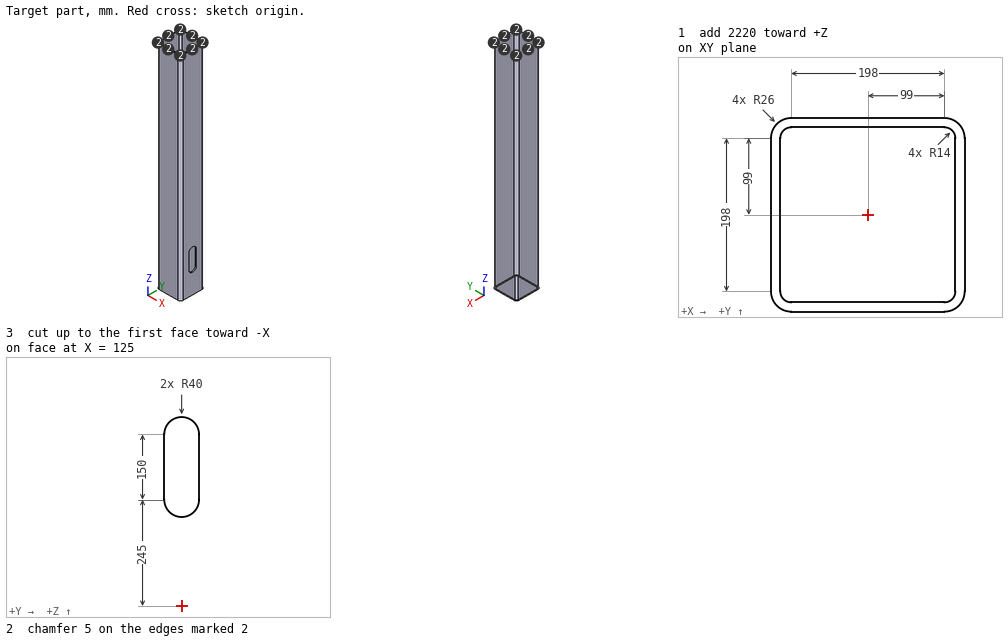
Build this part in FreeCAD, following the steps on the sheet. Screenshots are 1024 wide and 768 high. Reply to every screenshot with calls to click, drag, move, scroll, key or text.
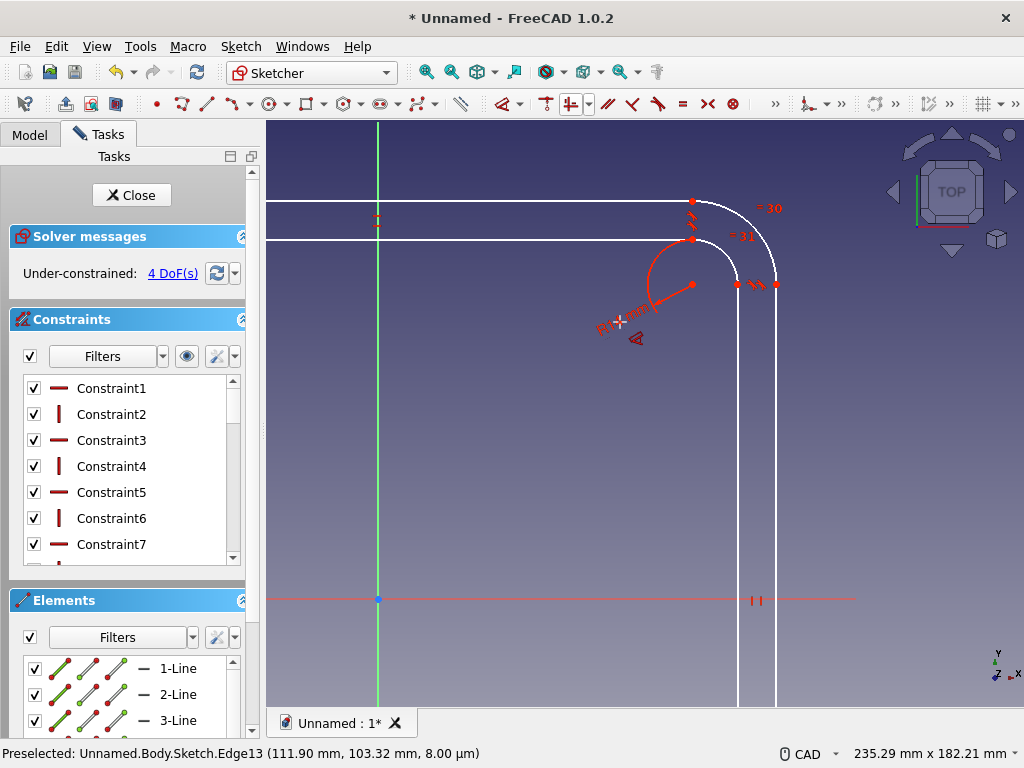
click(503, 201)
click(493, 167)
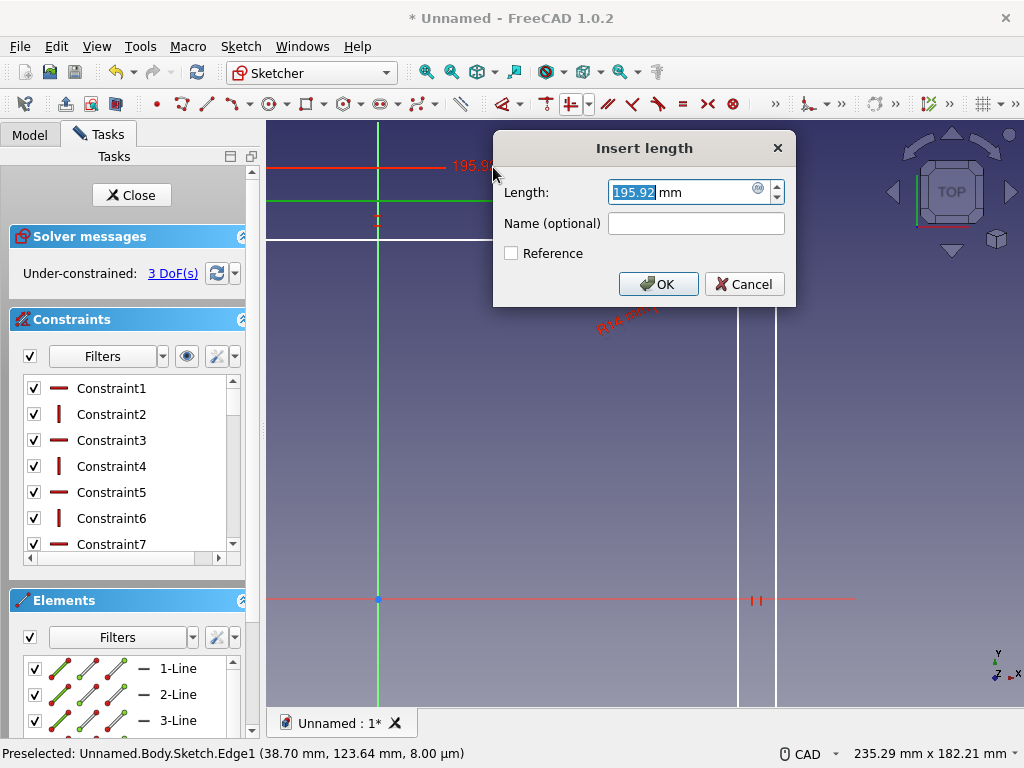
text(198)
key(Return)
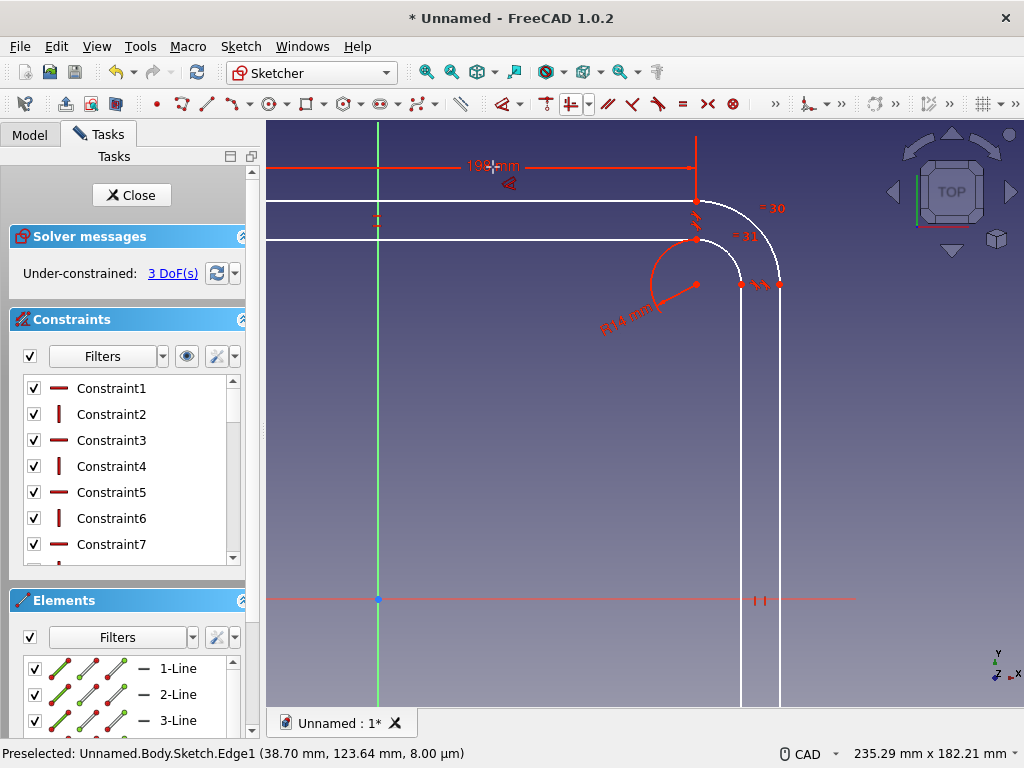
scroll(738, 262, down, 4)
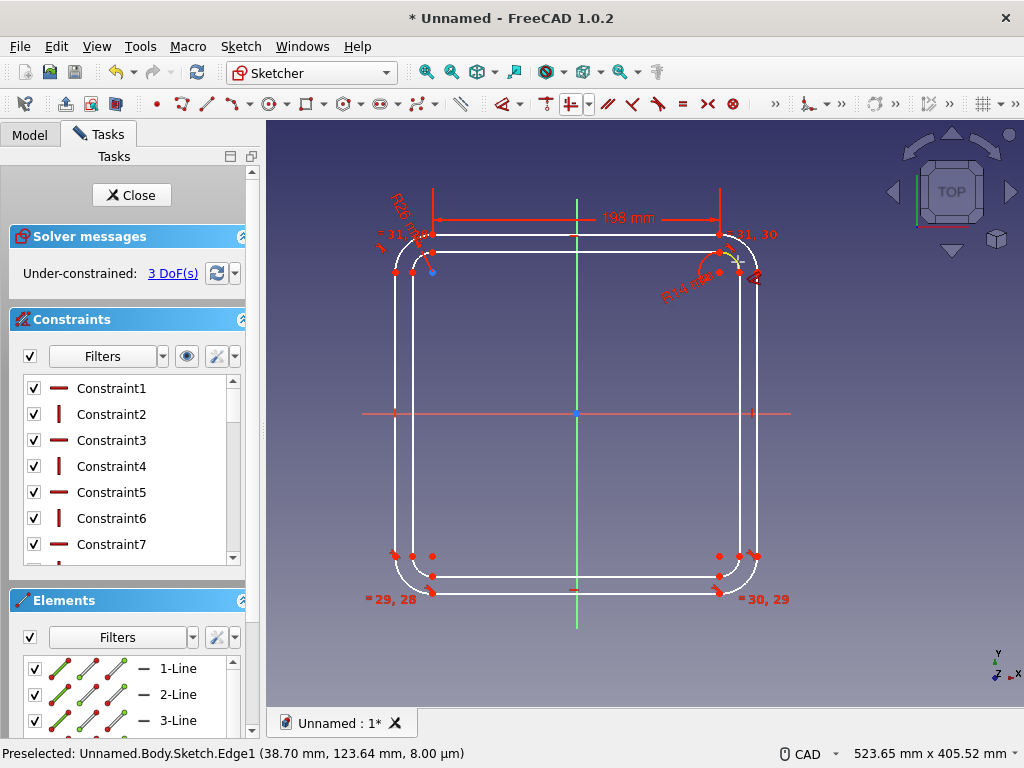
click(395, 358)
click(361, 349)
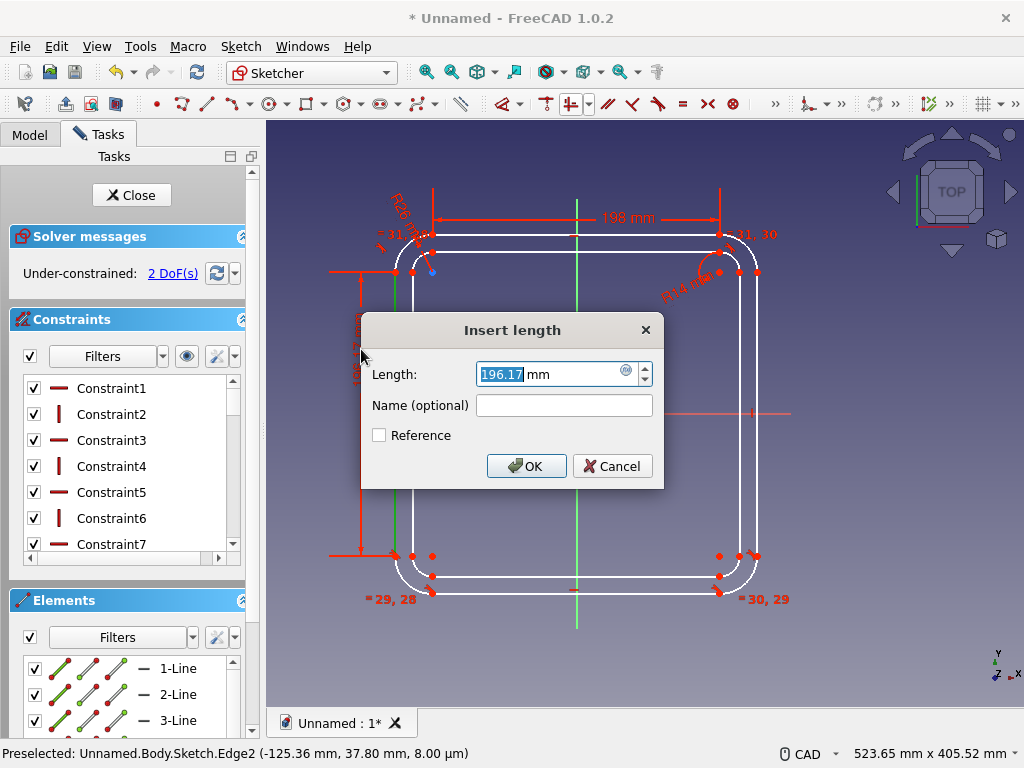
text(198)
key(Return)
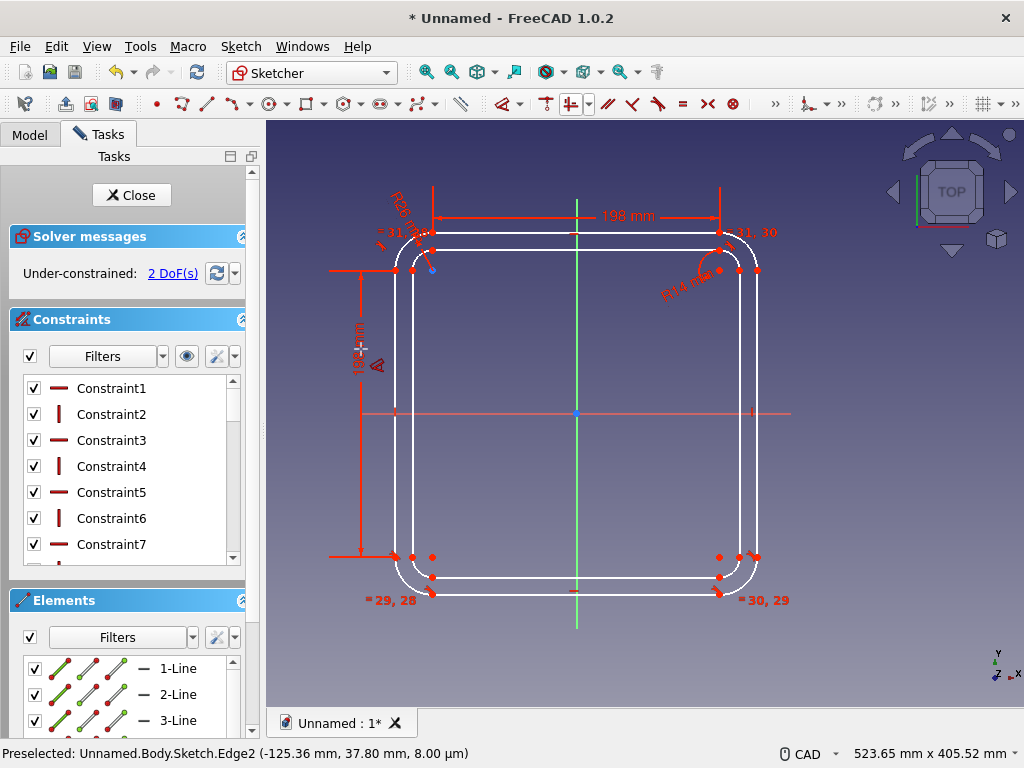
click(720, 233)
click(648, 199)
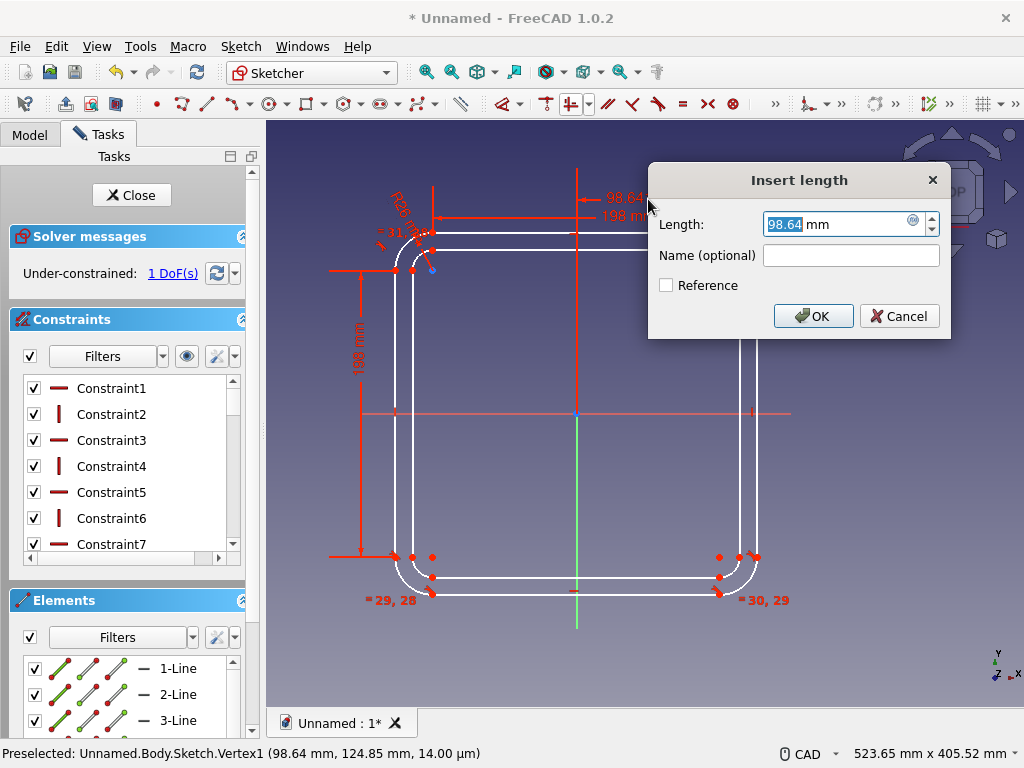
text(99)
key(Return)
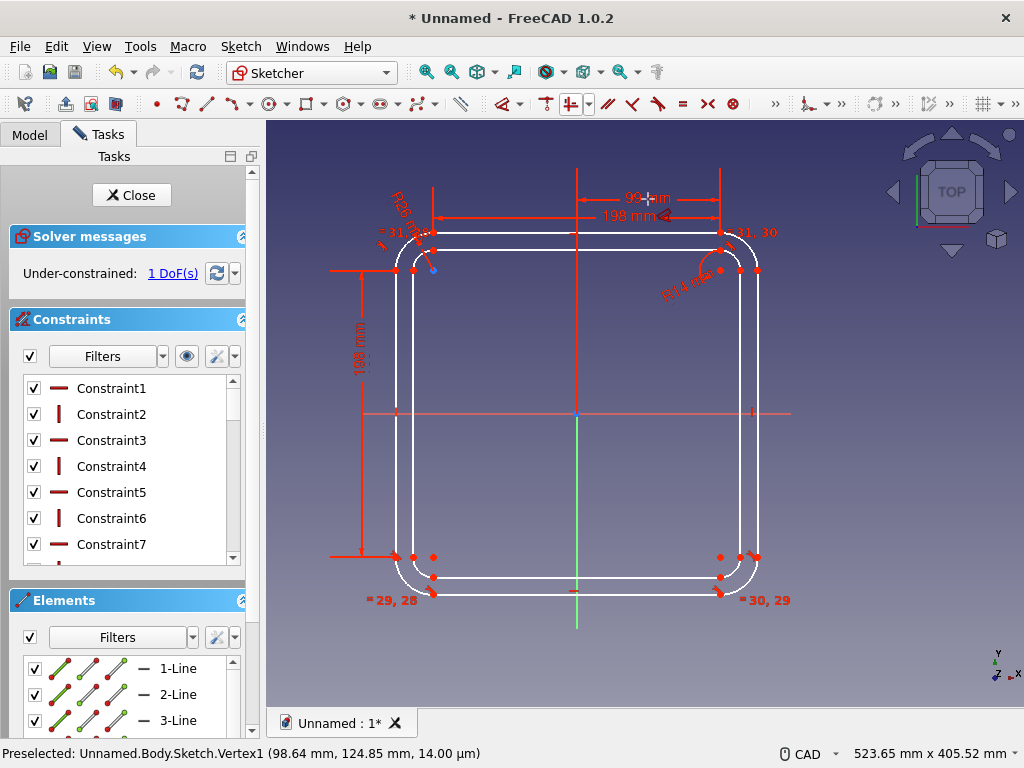
click(396, 271)
click(362, 309)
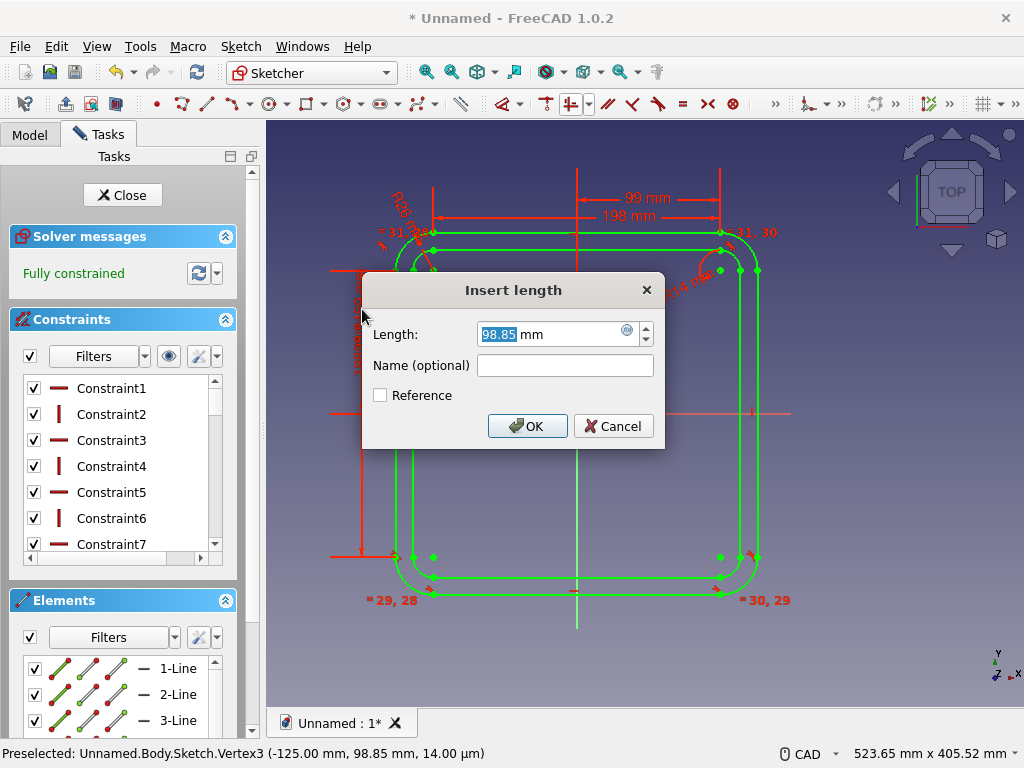
text(99)
key(Return)
key(Escape)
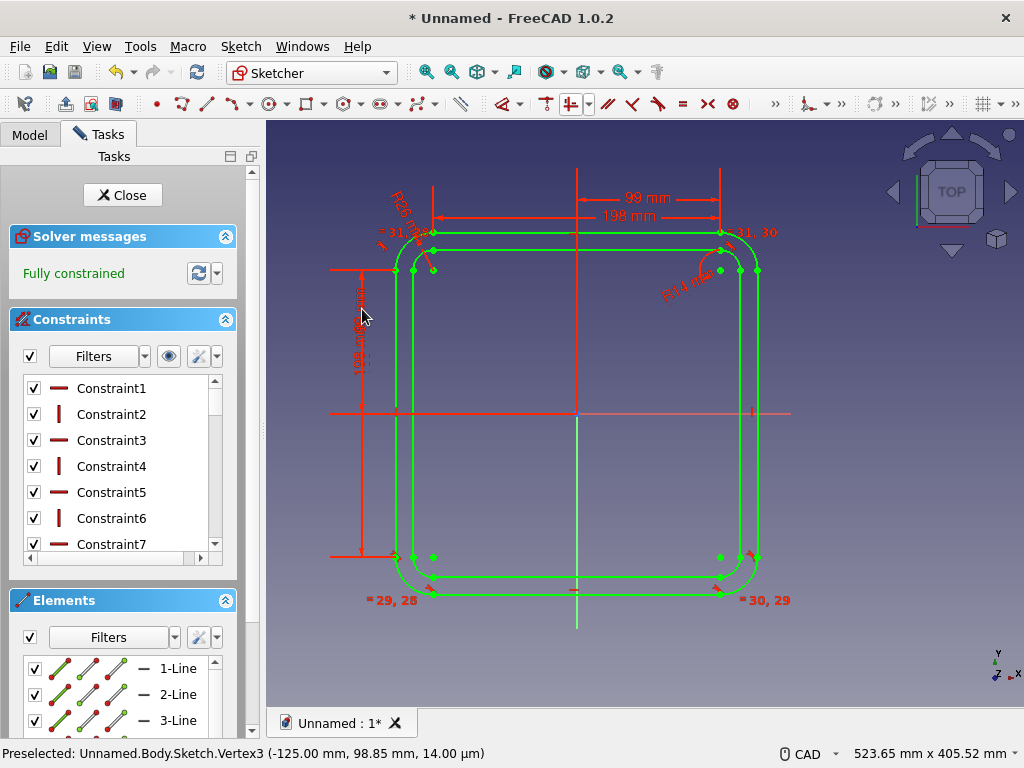
click(123, 195)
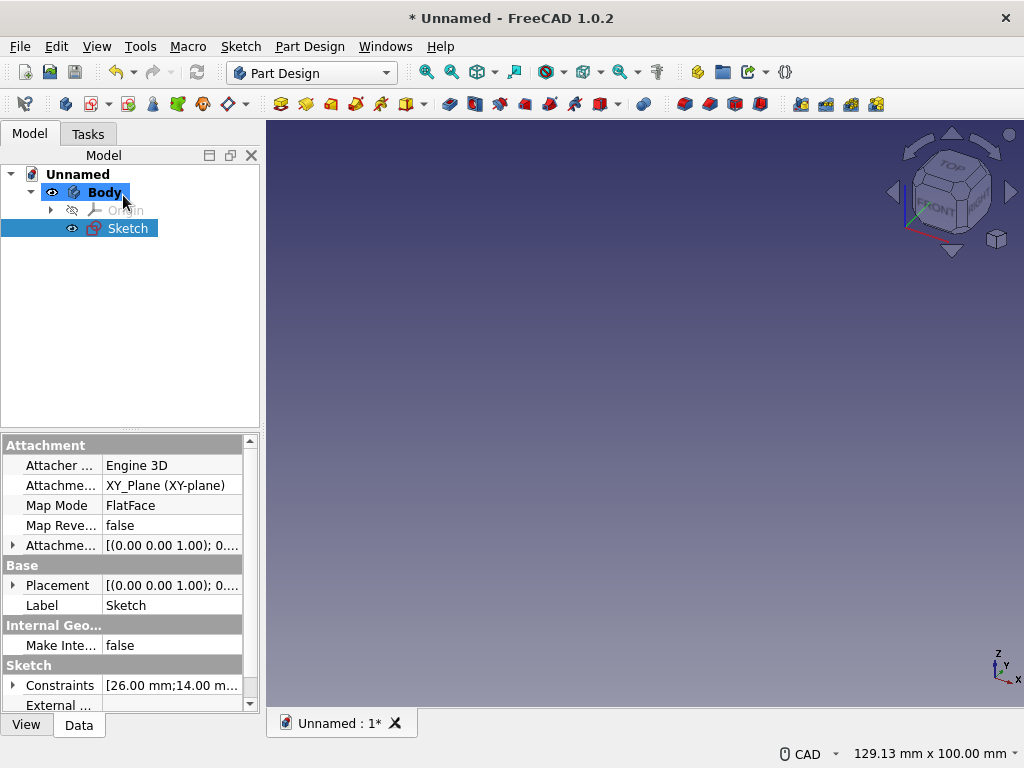
click(281, 104)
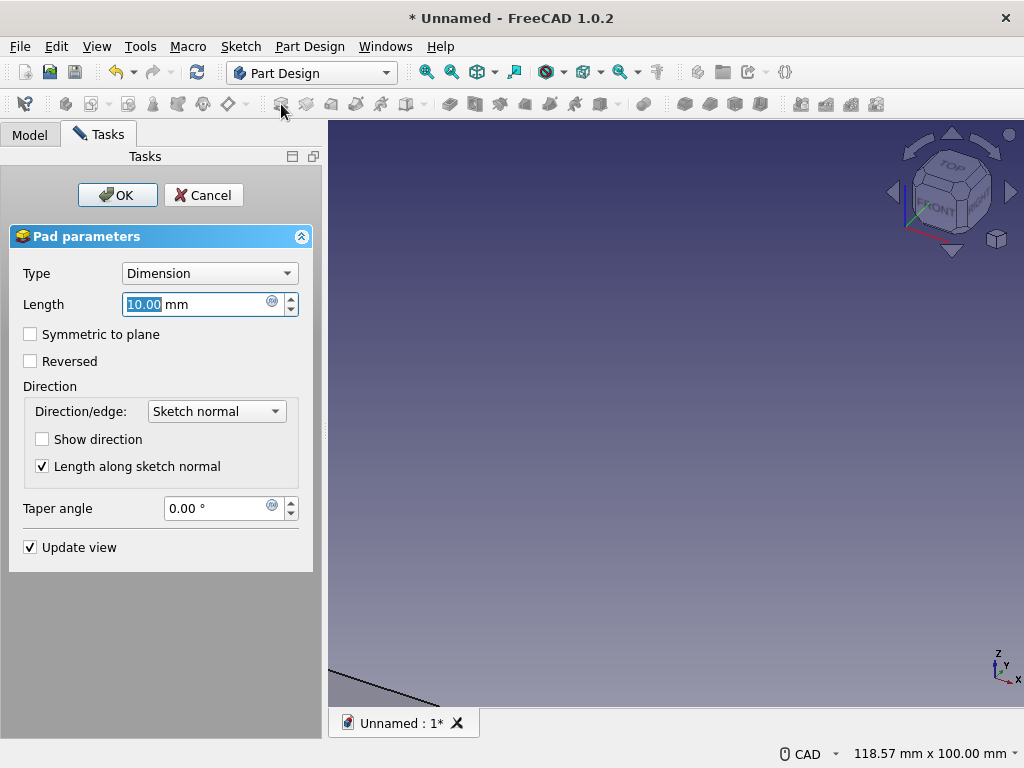
text(2220)
key(Tab)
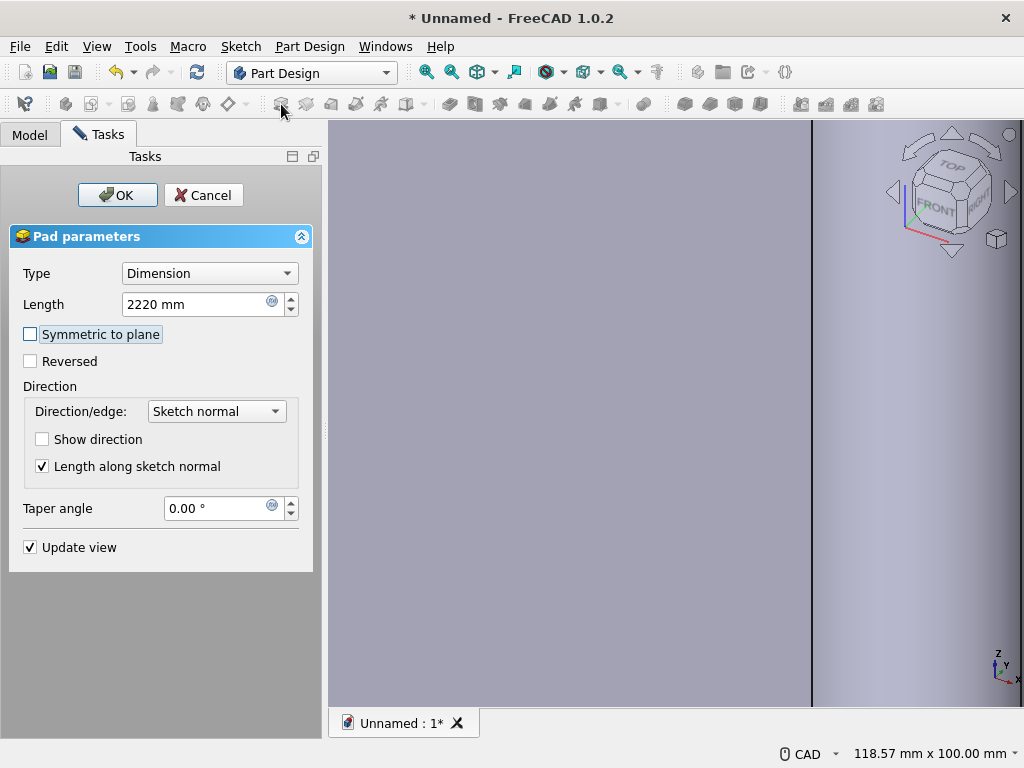
click(118, 195)